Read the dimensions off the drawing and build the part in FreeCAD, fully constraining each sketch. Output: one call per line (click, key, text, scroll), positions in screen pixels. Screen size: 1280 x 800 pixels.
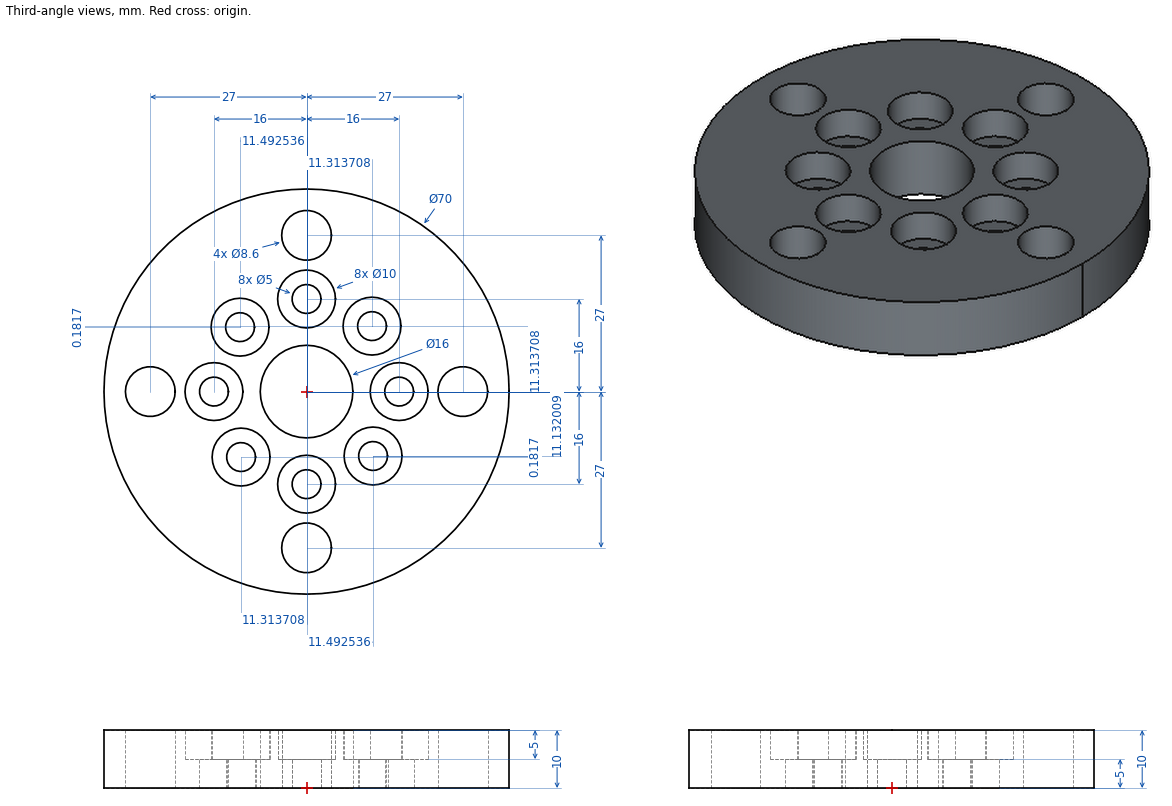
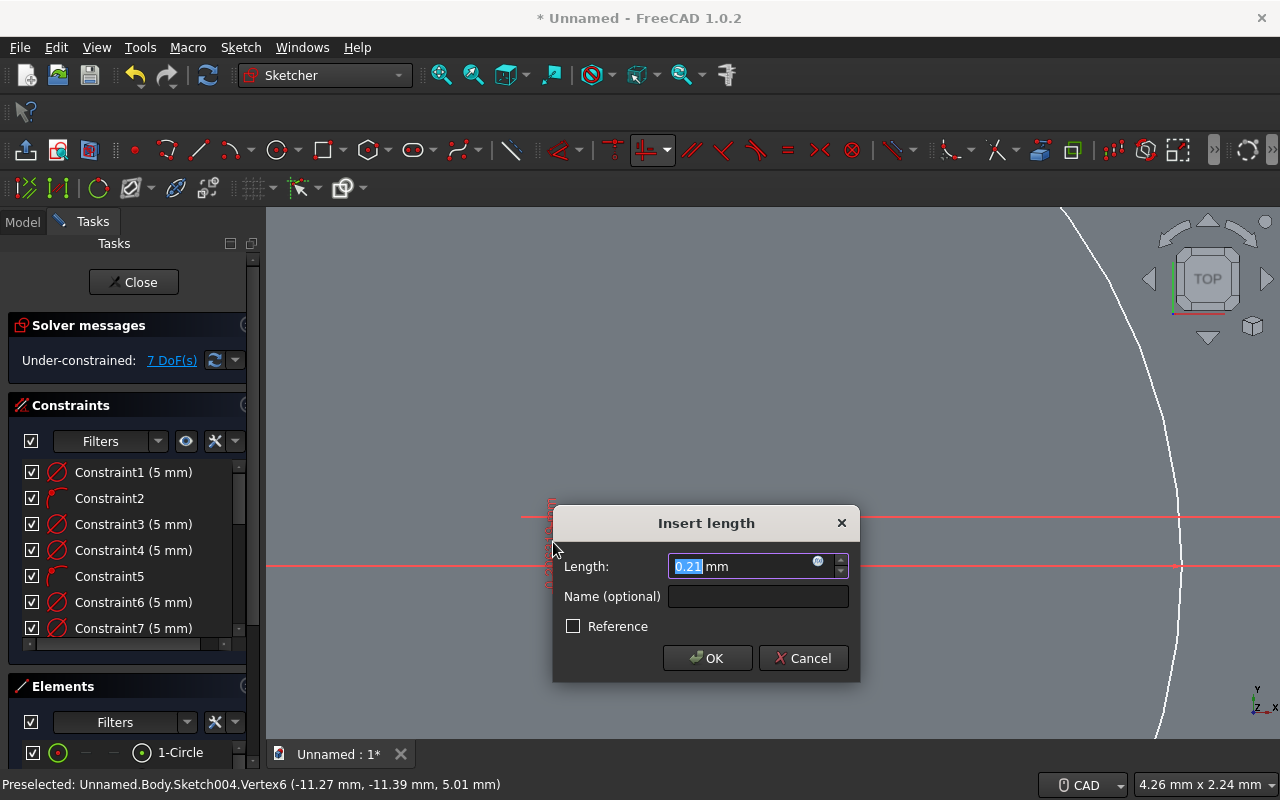
text(0.1817)
key(Return)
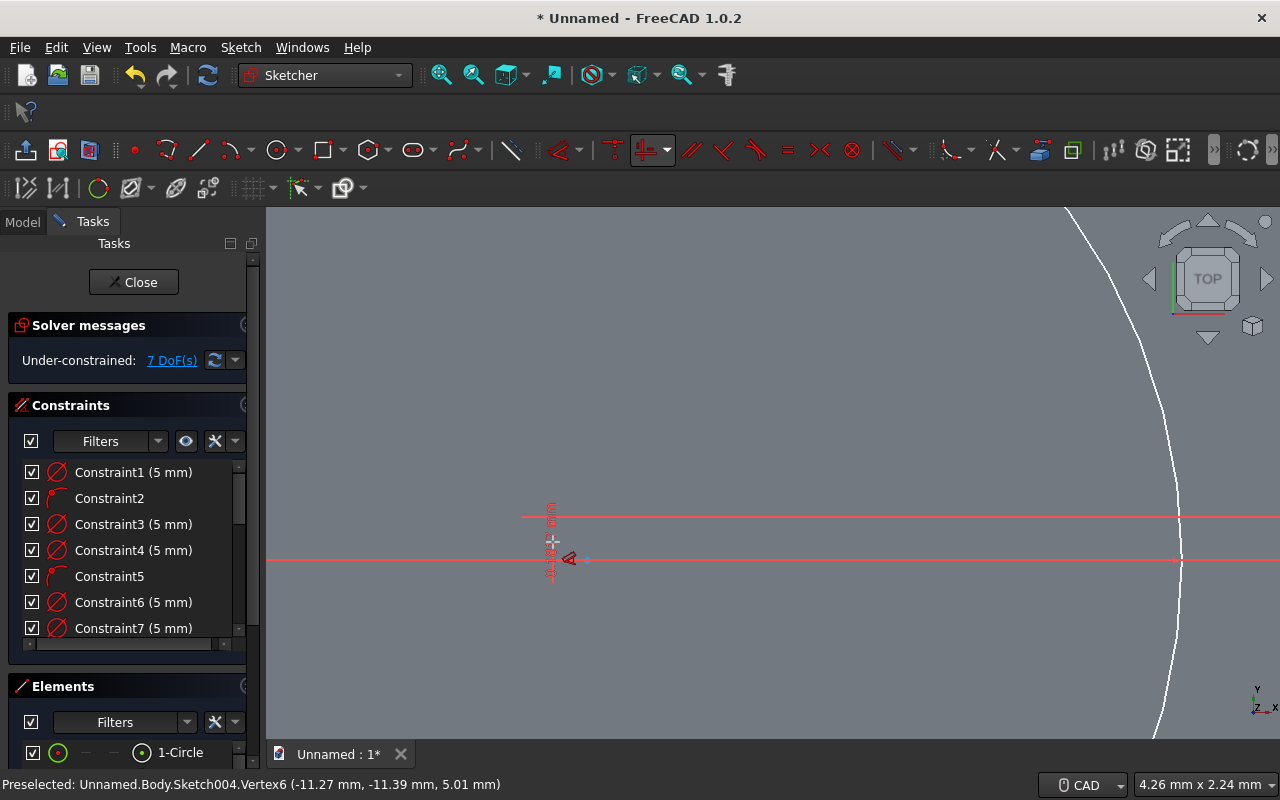
scroll(596, 584, down, 16)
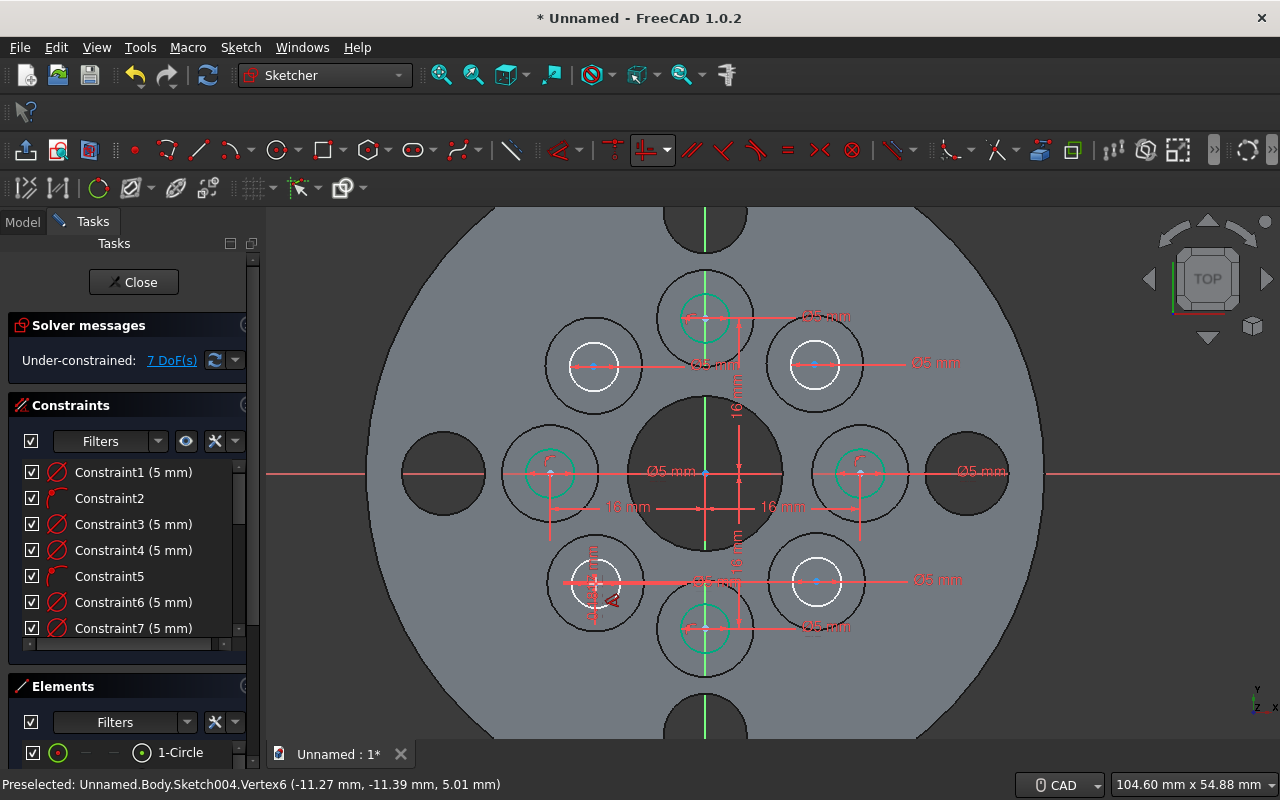
scroll(815, 365, up, 16)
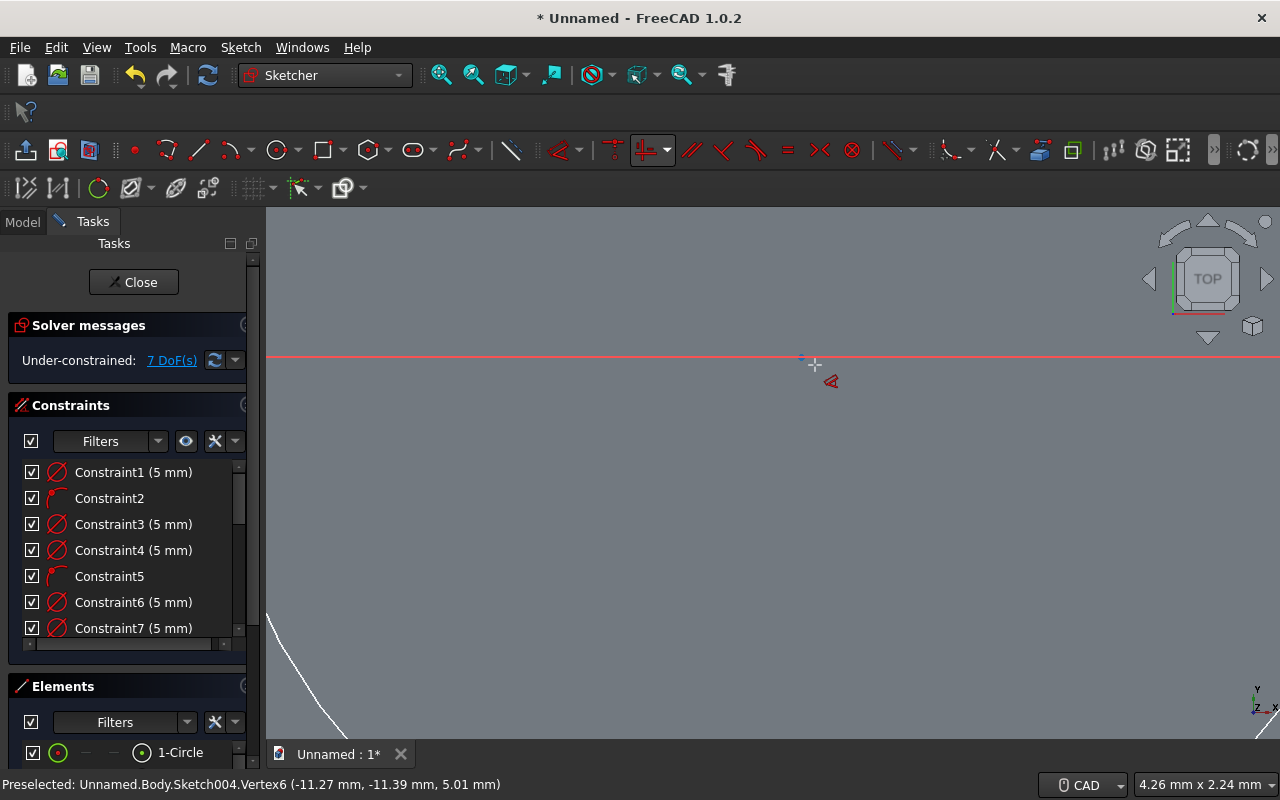
click(801, 357)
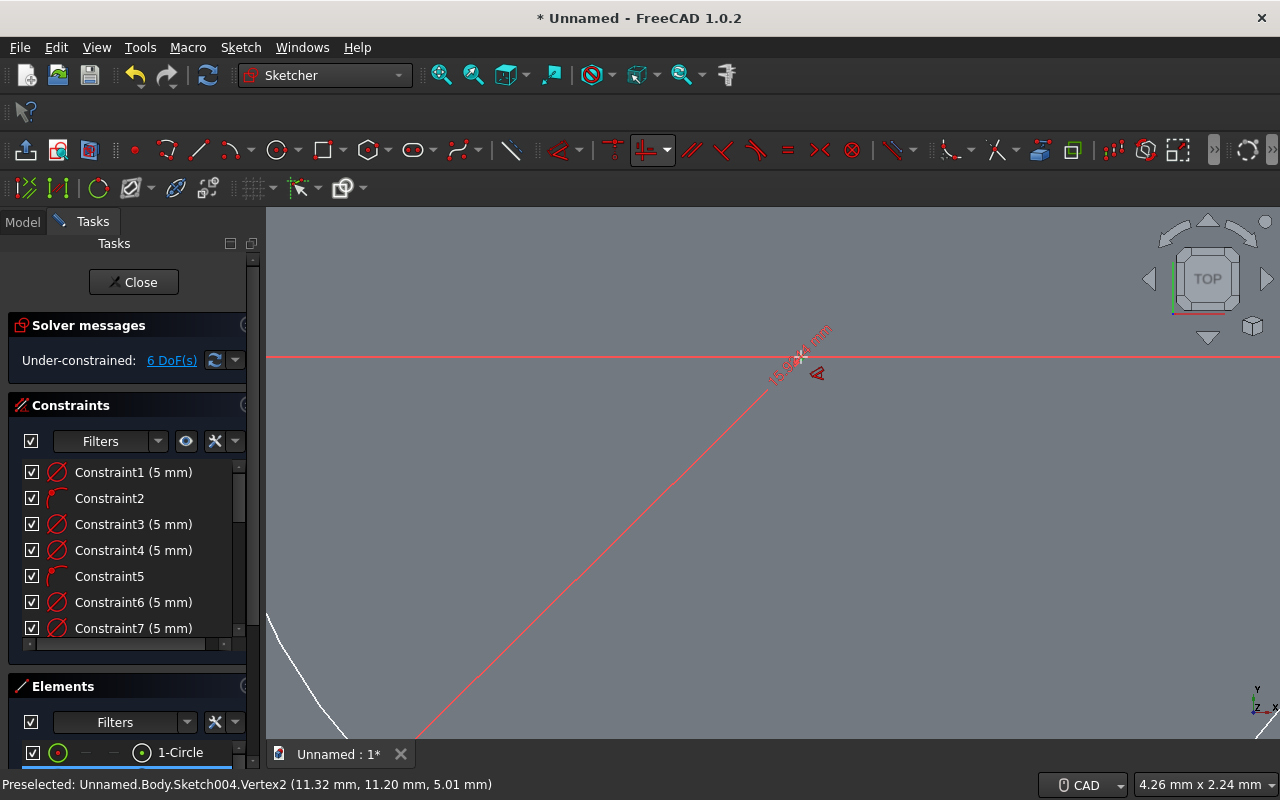
scroll(815, 365, down, 16)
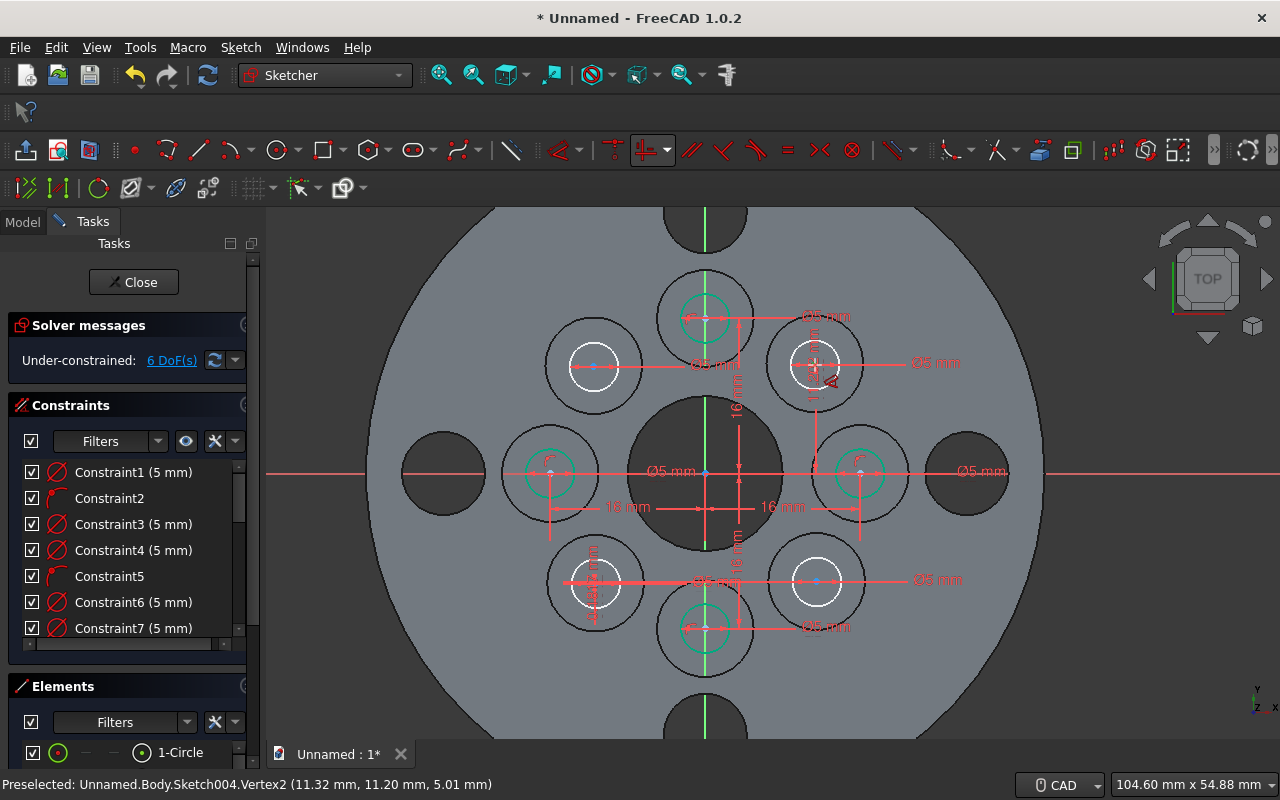
scroll(594, 367, up, 16)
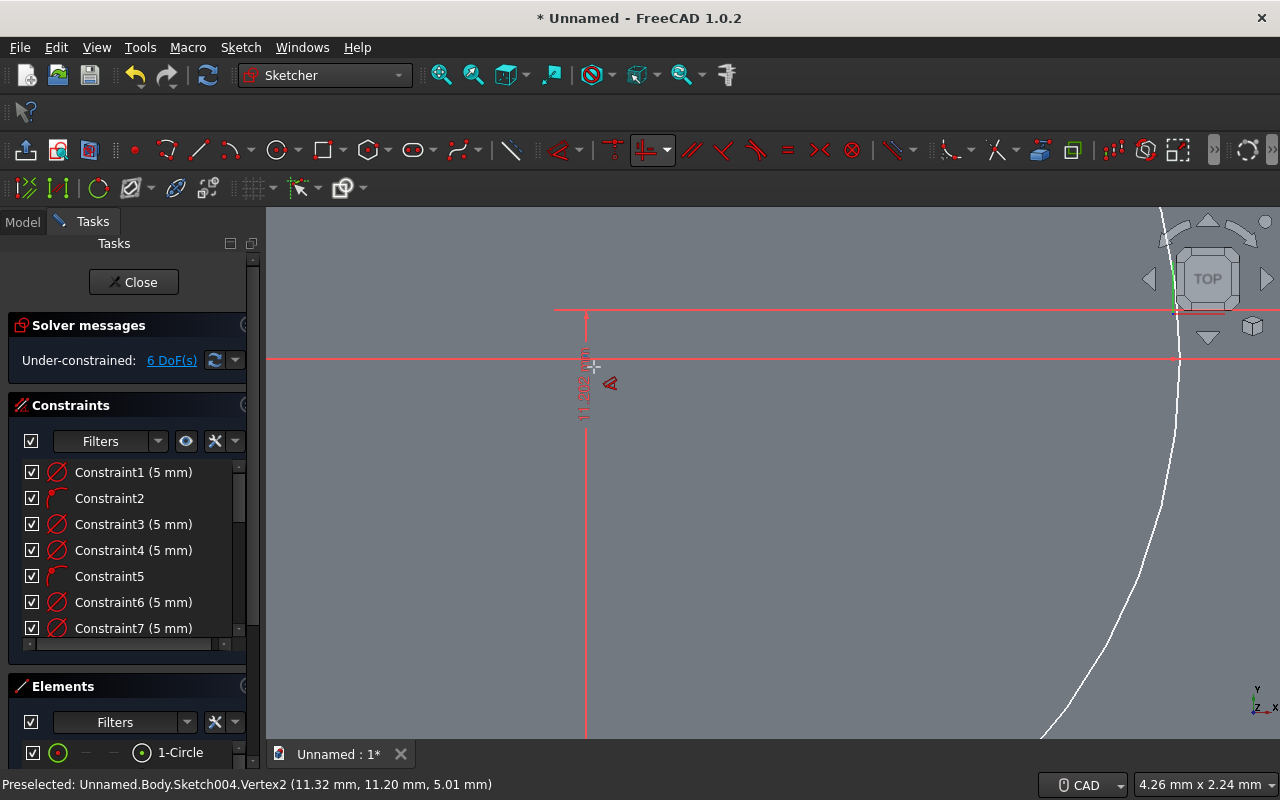
click(585, 359)
click(551, 334)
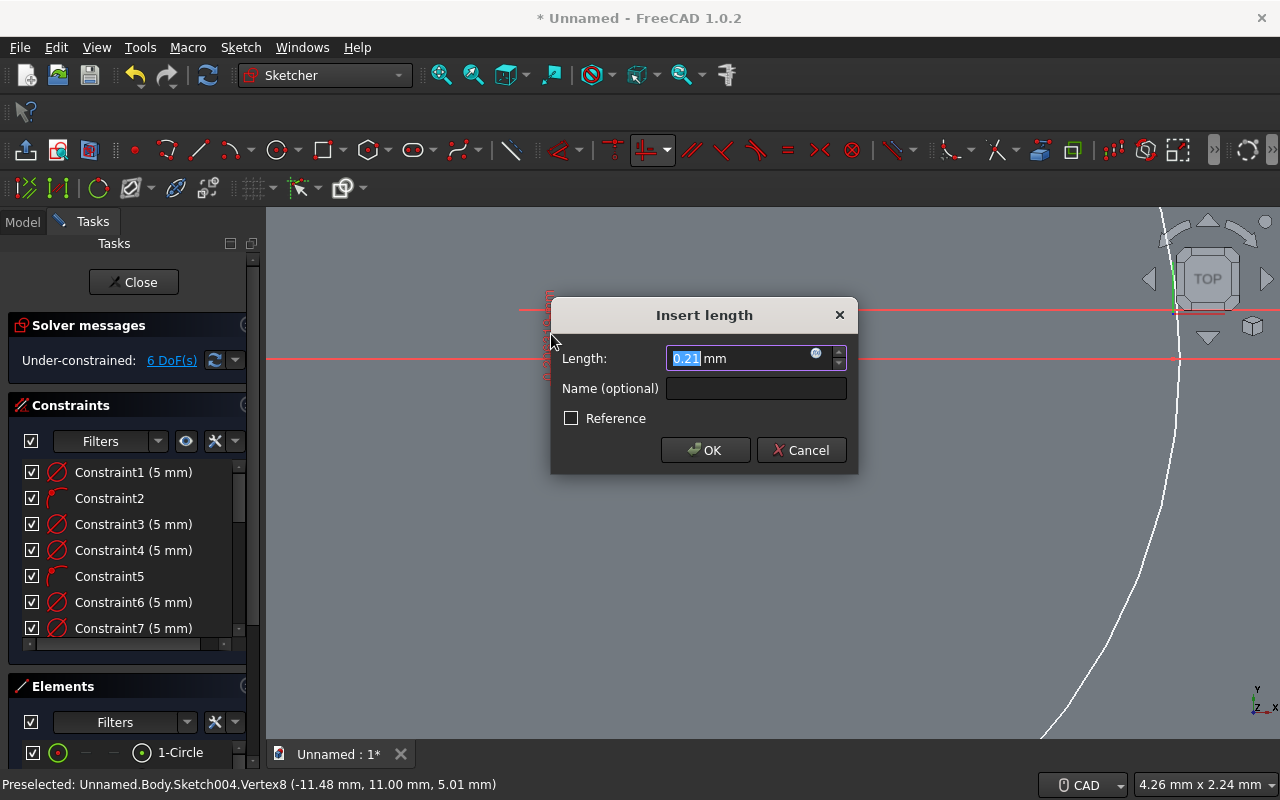
text(0.1817)
key(Return)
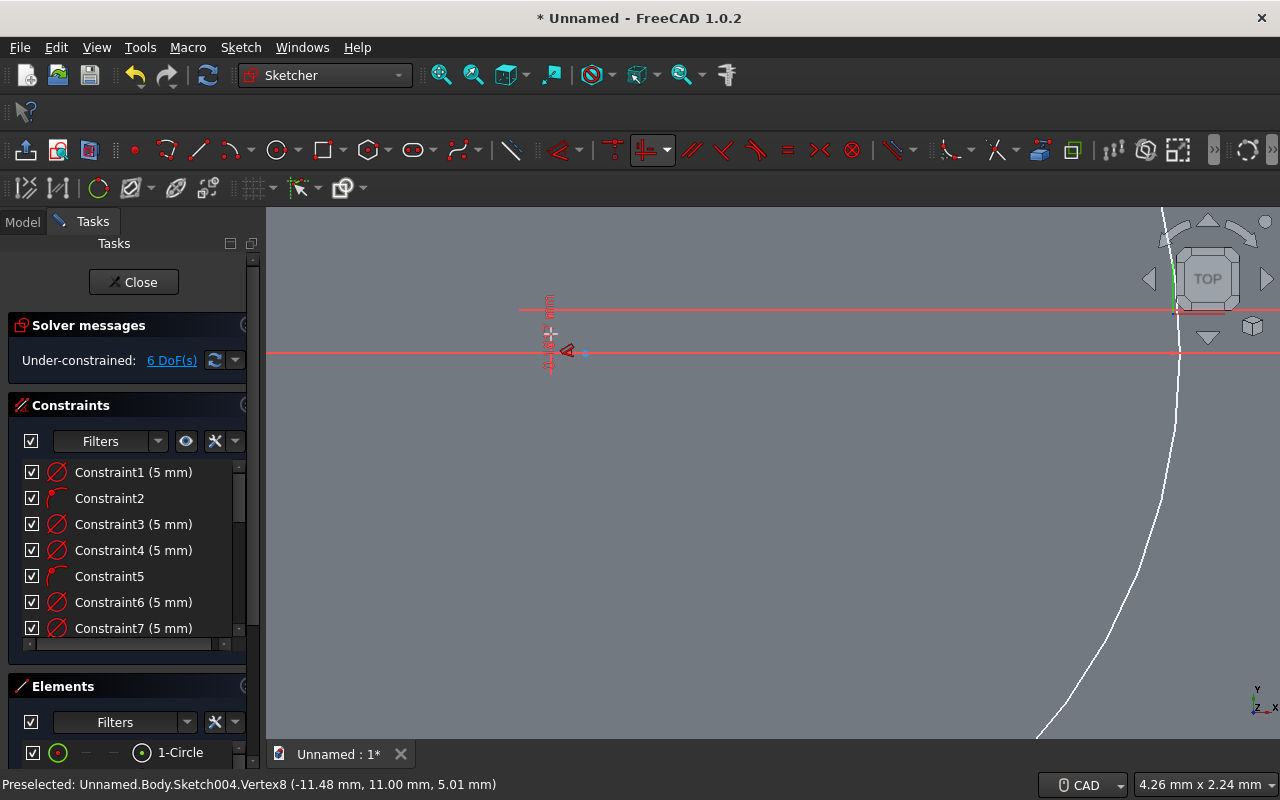
scroll(594, 367, down, 16)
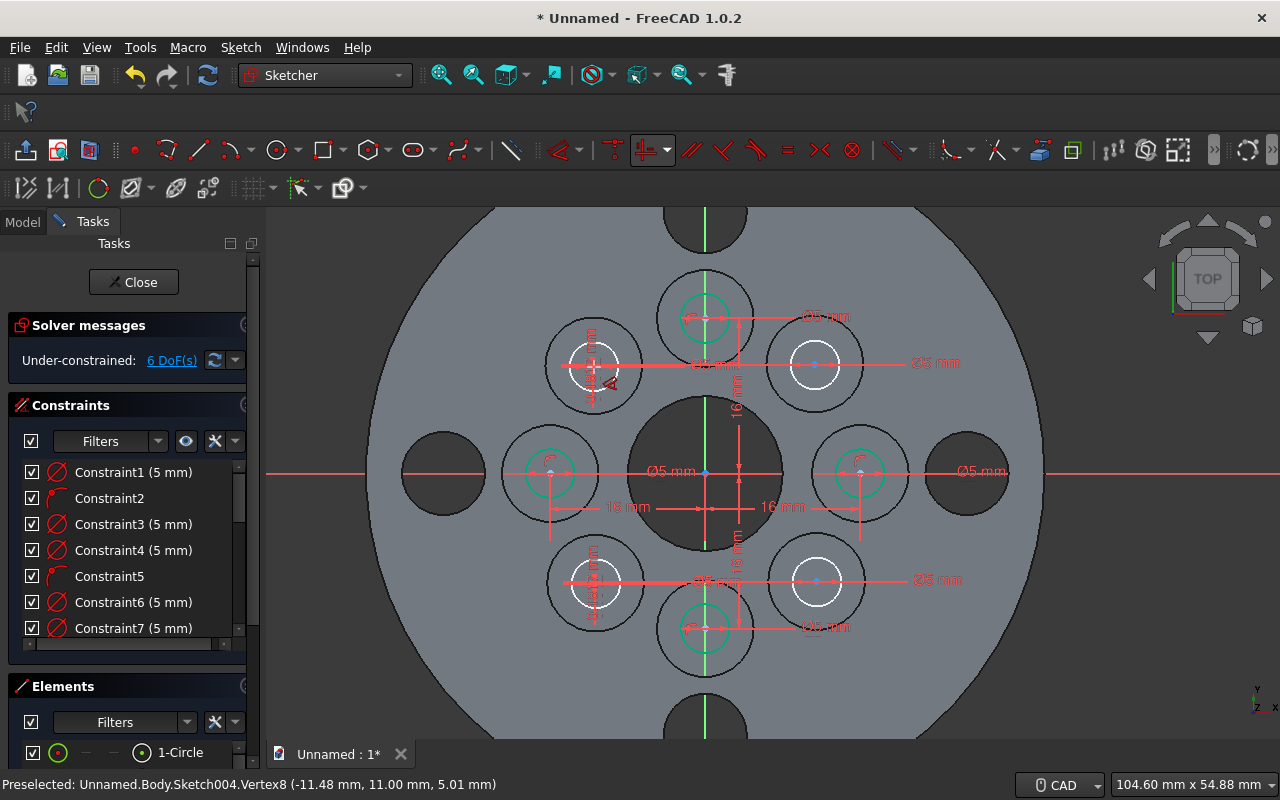
click(815, 365)
click(760, 331)